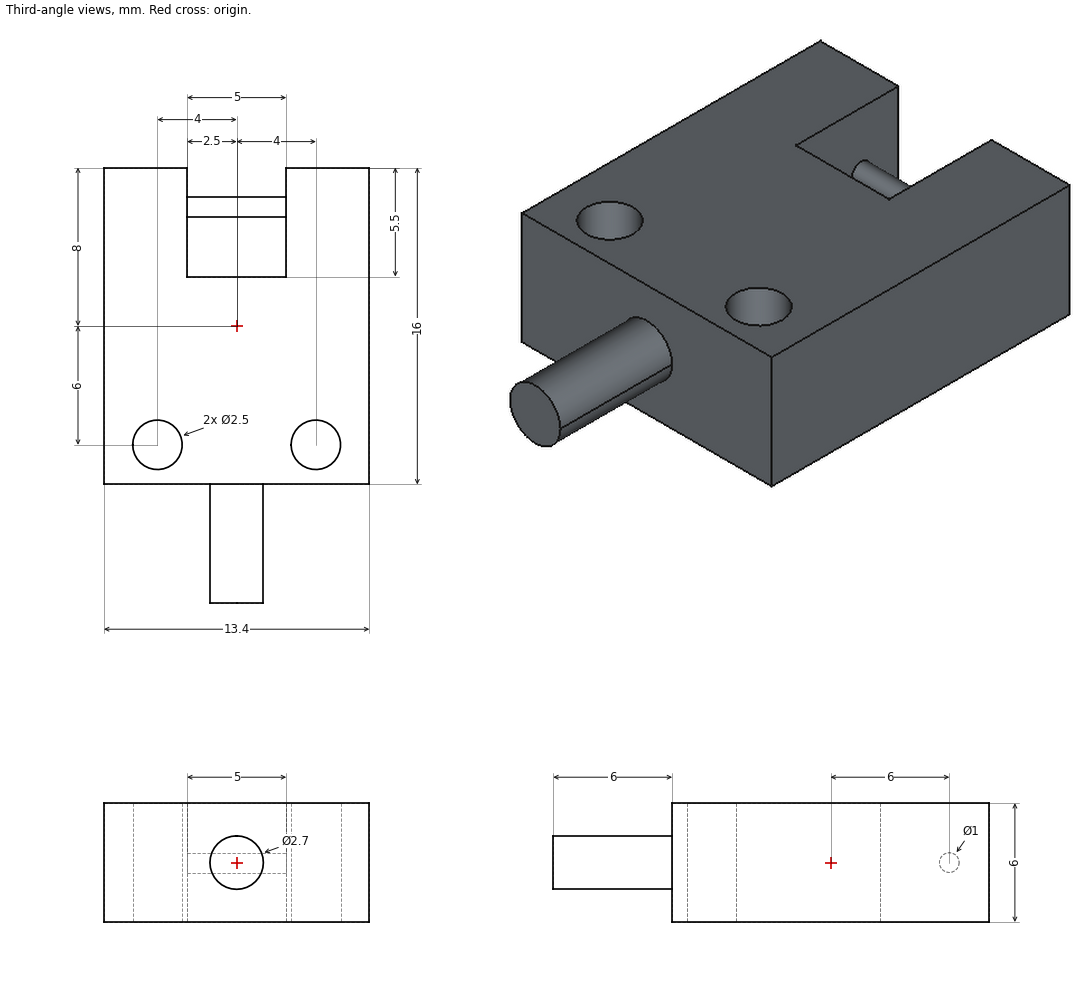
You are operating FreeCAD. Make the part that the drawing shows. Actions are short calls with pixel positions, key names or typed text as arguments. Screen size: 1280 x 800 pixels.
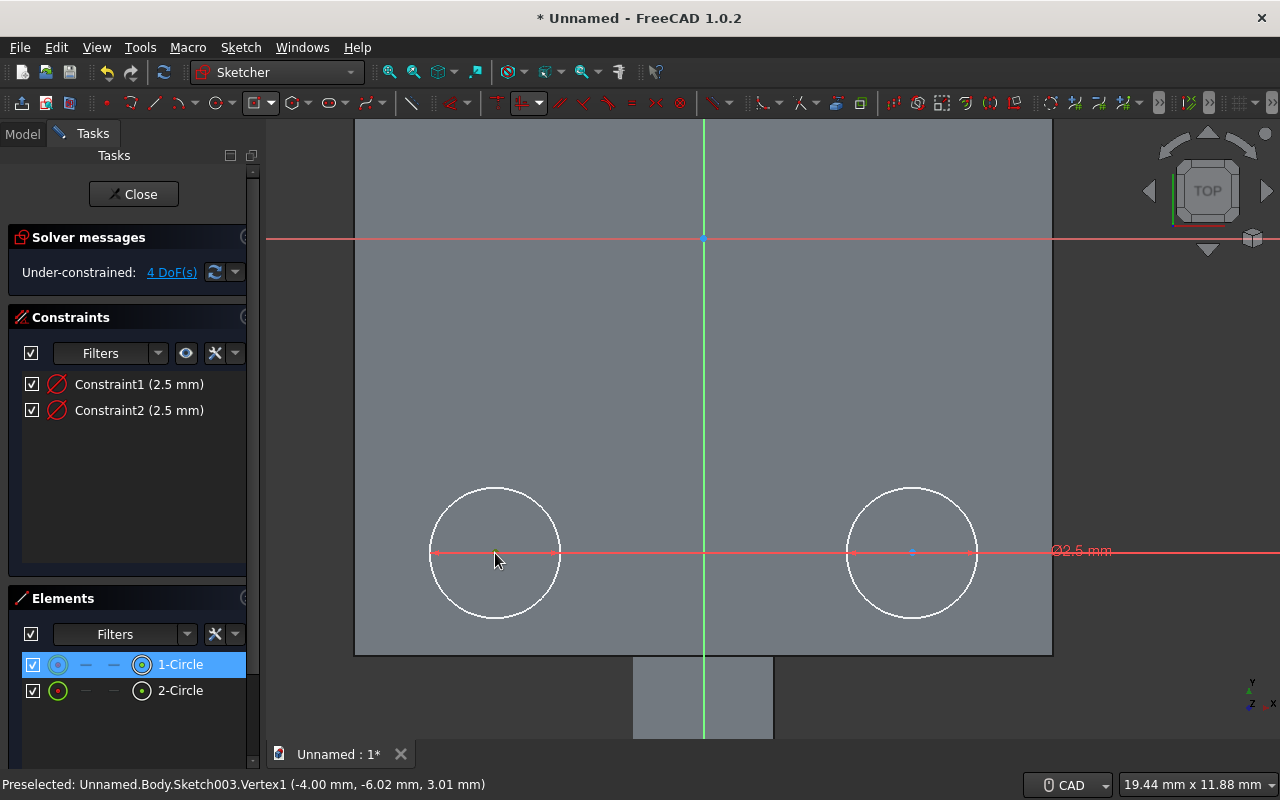
click(912, 553)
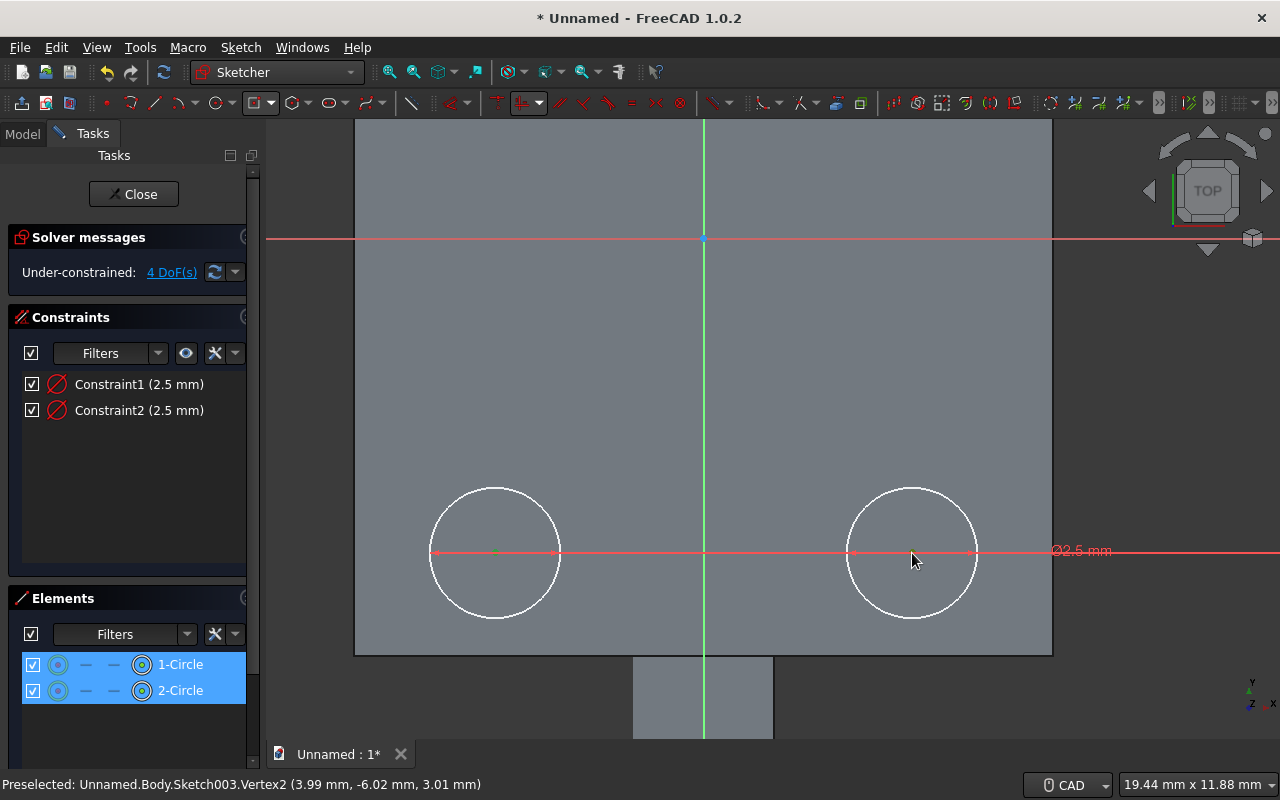
key(h)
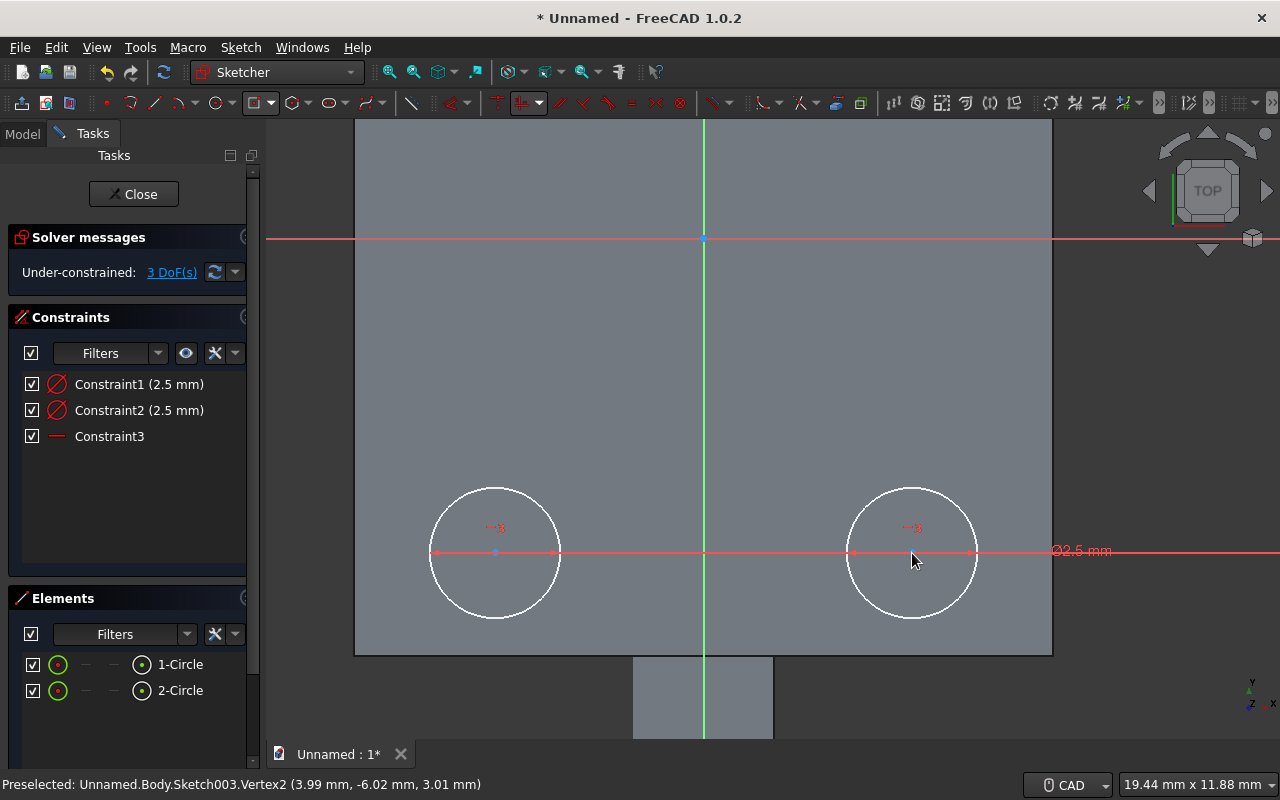
key(d)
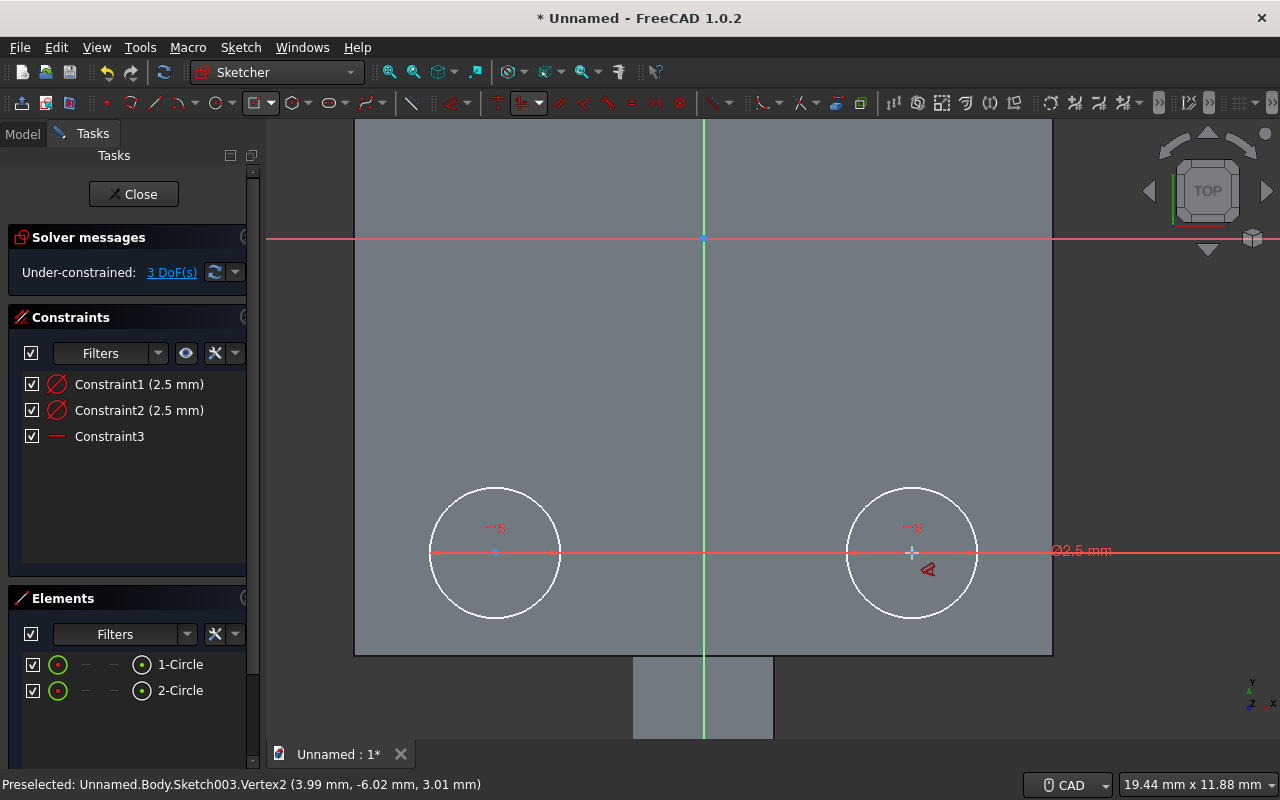
click(495, 553)
click(599, 205)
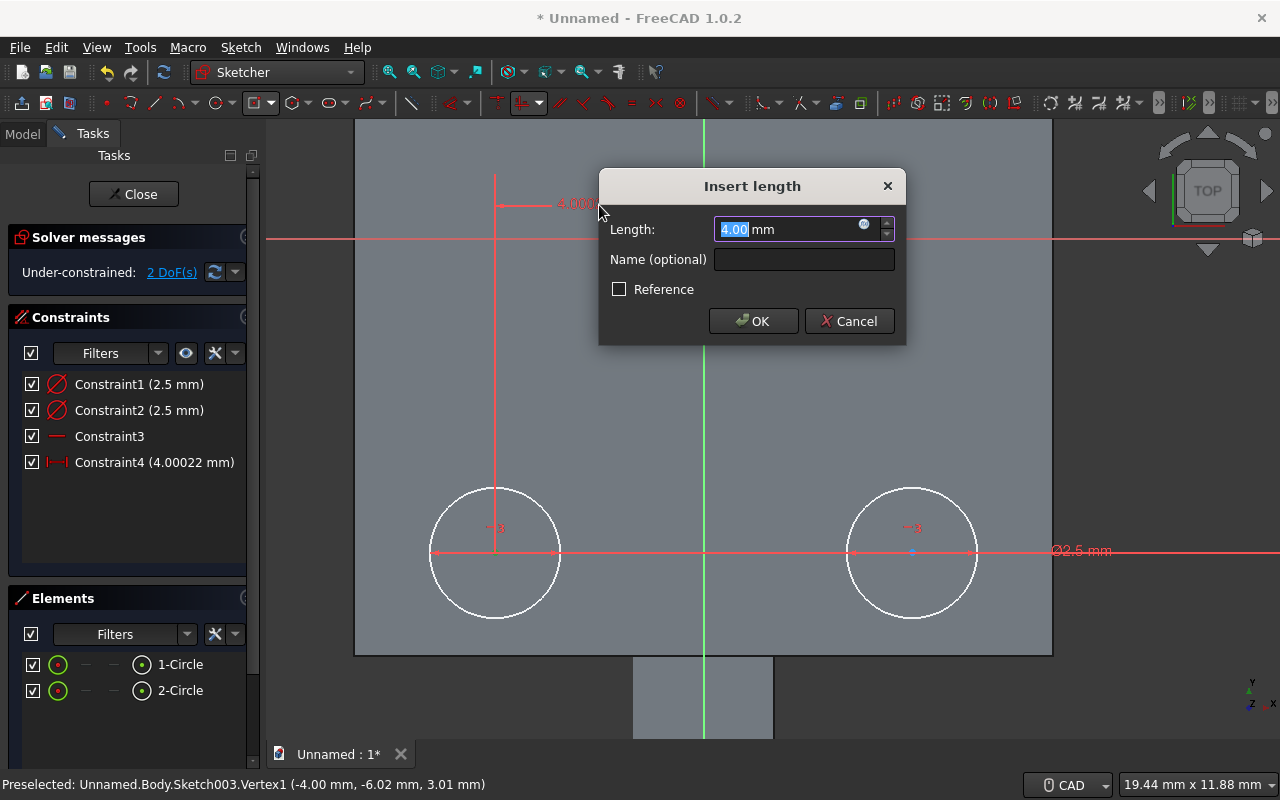
text(4)
key(Return)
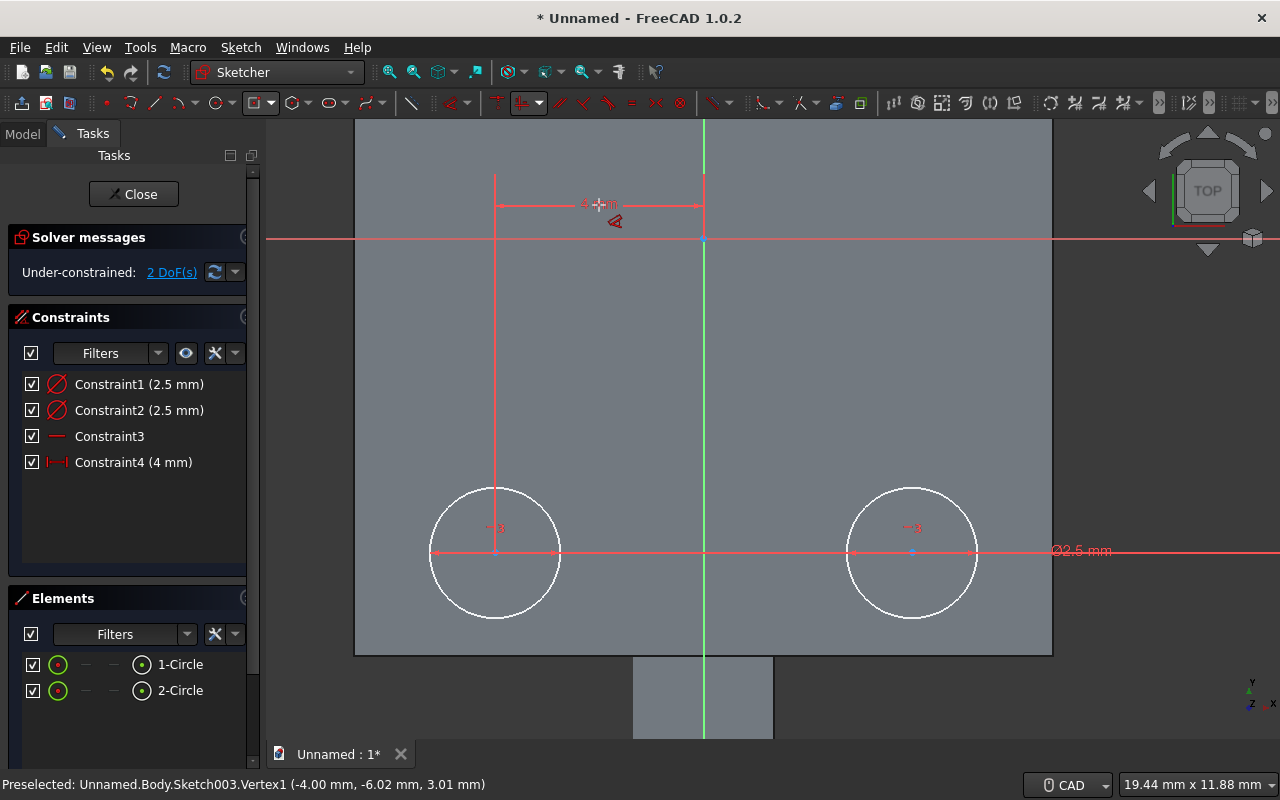
click(495, 553)
click(461, 396)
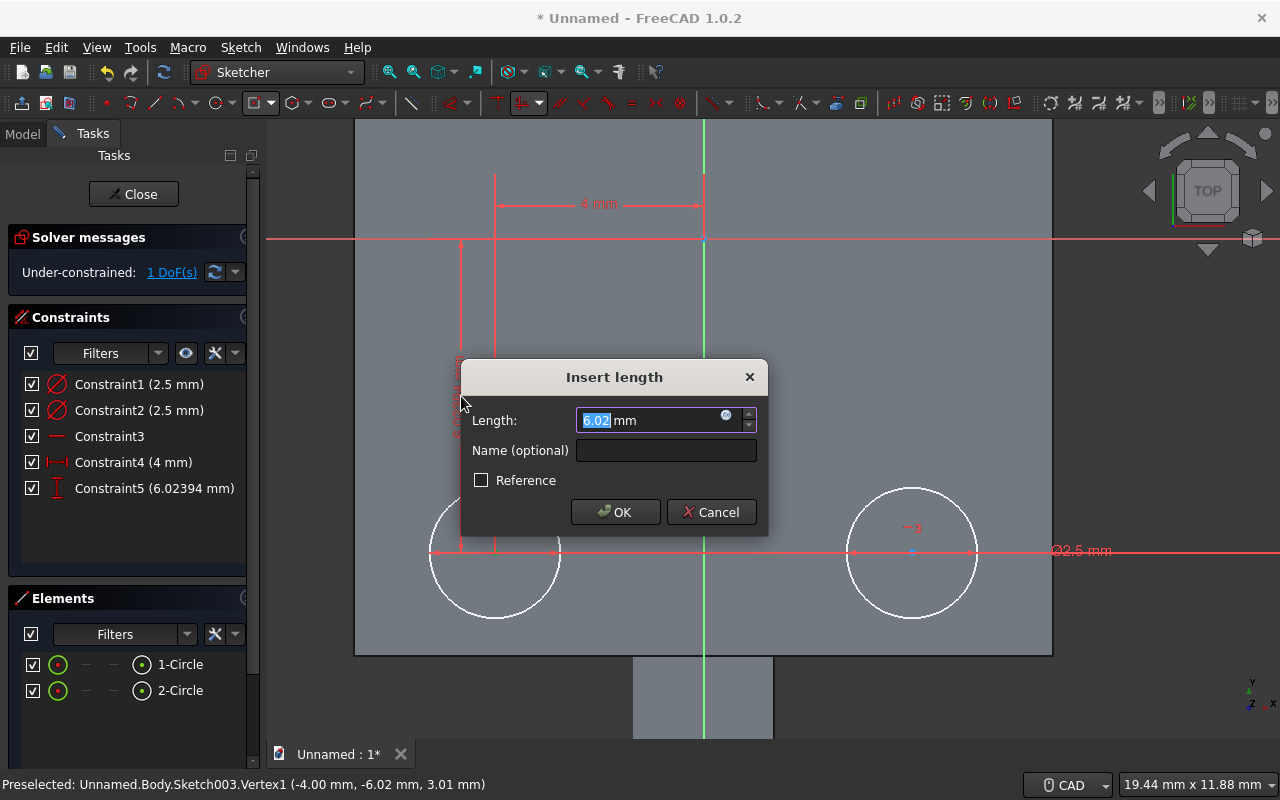
text(6)
key(Return)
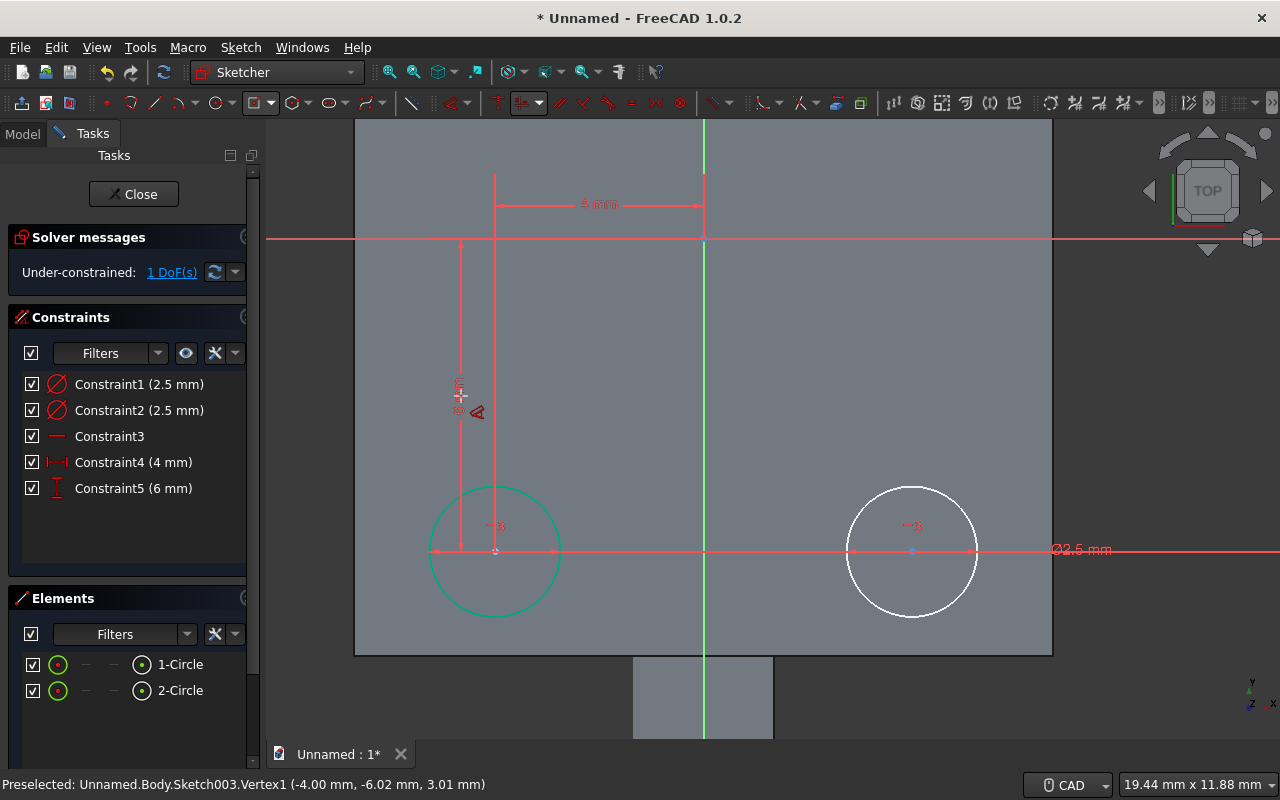
click(912, 552)
click(808, 205)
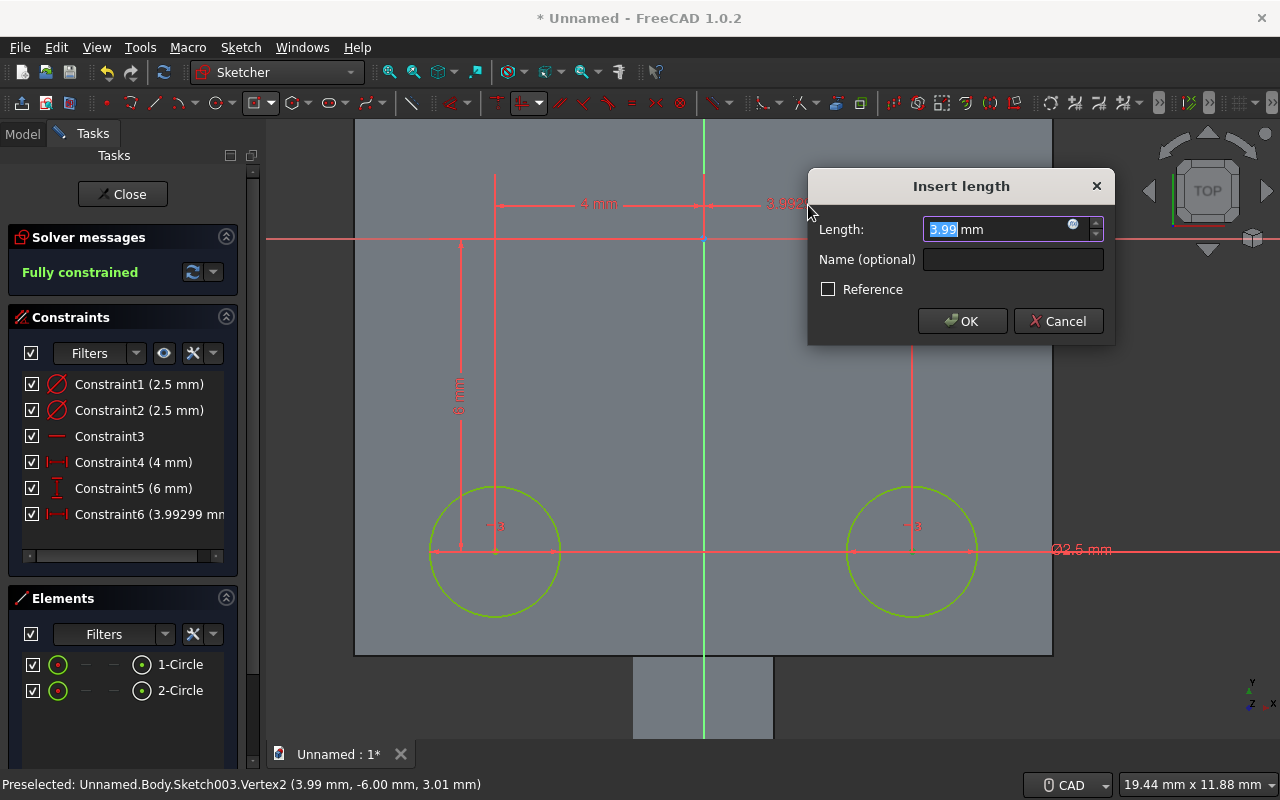
text(4)
key(Return)
key(Escape)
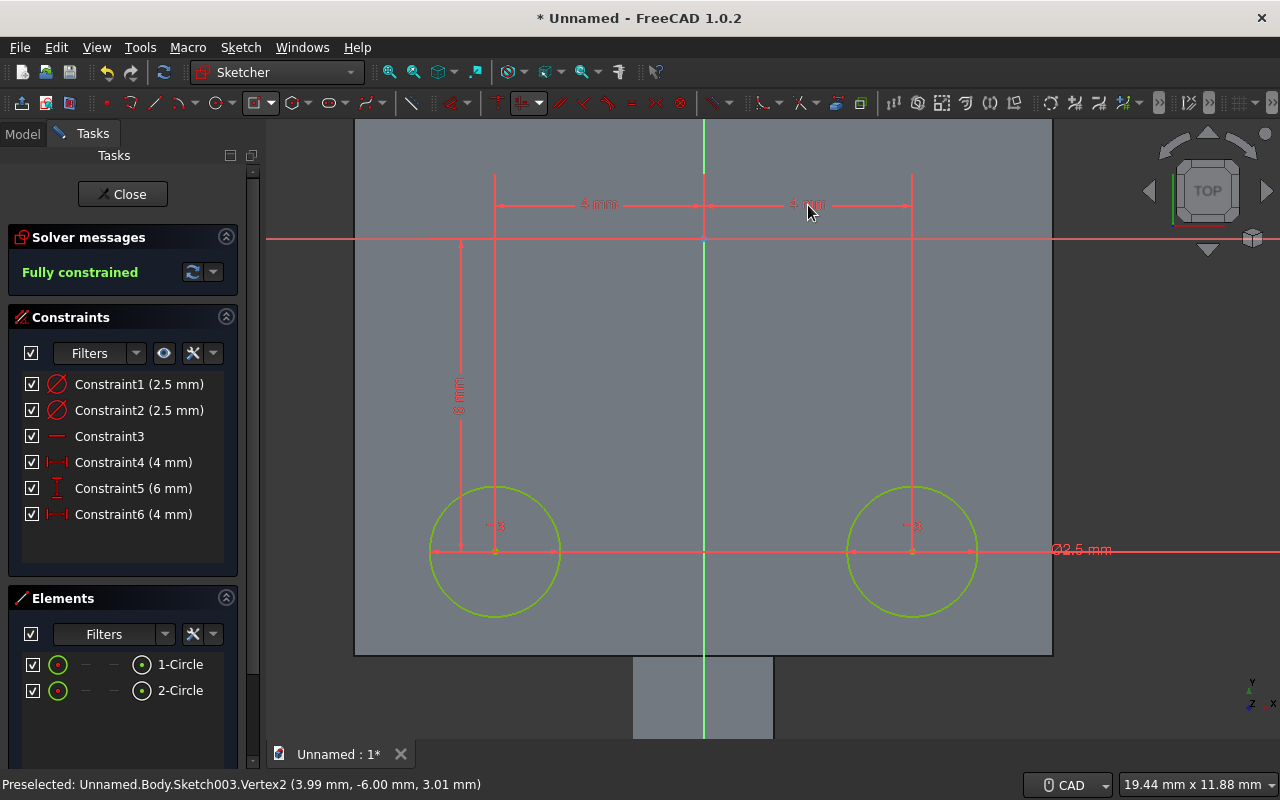
click(123, 194)